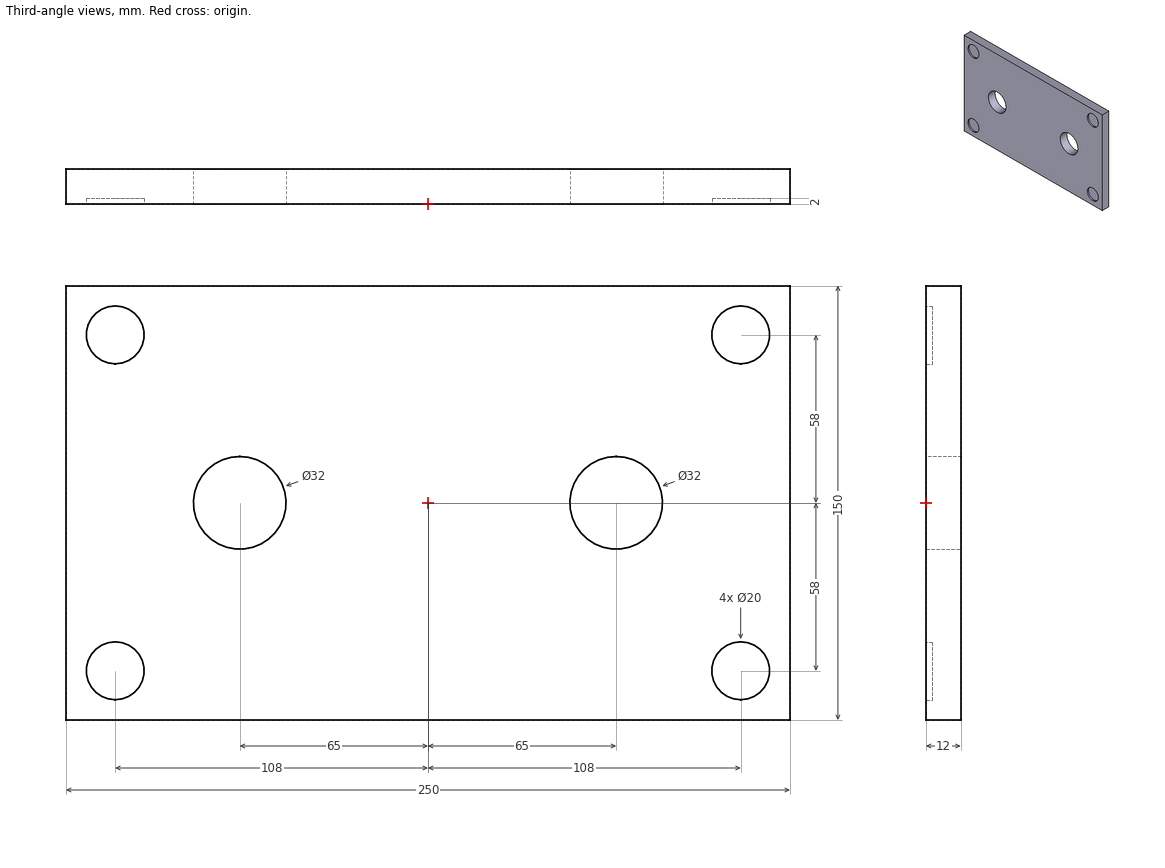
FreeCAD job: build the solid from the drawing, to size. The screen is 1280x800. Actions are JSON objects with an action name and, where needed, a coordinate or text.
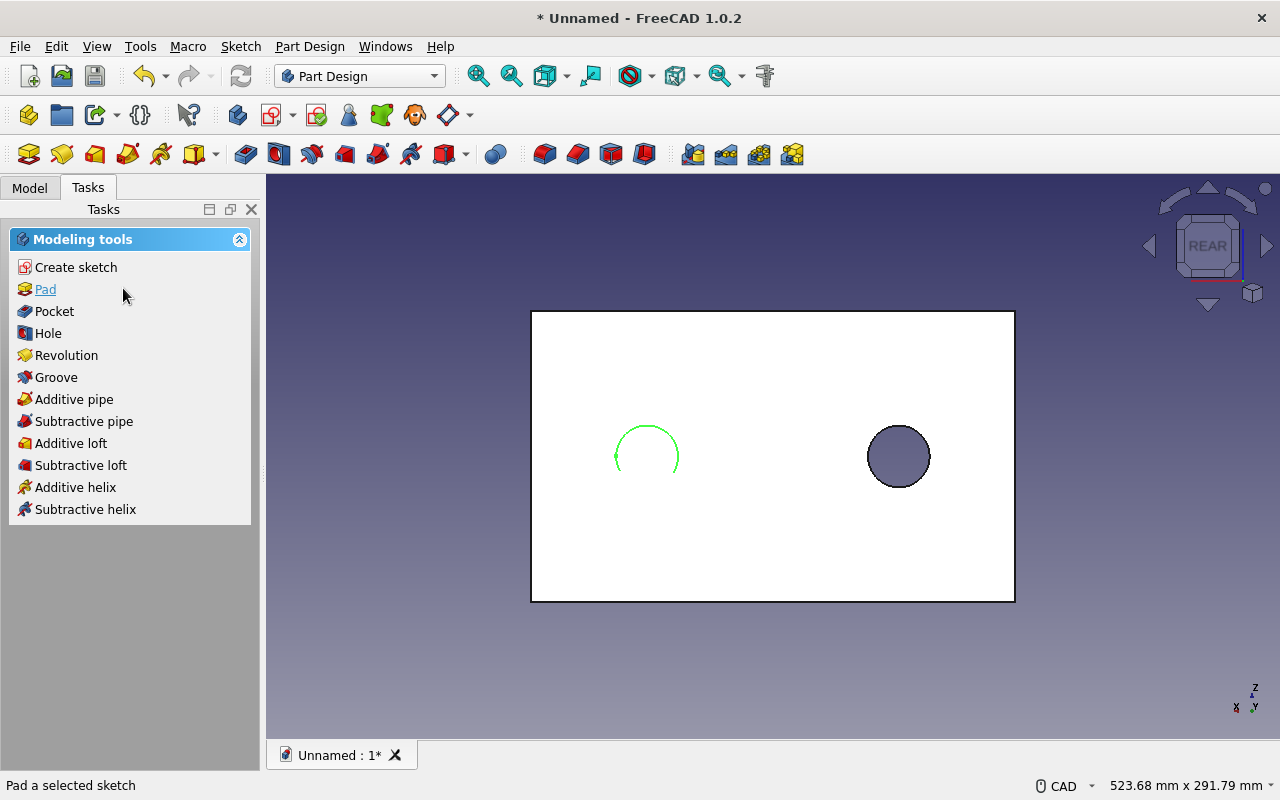
{"action": "left_click", "coordinate": [246, 154]}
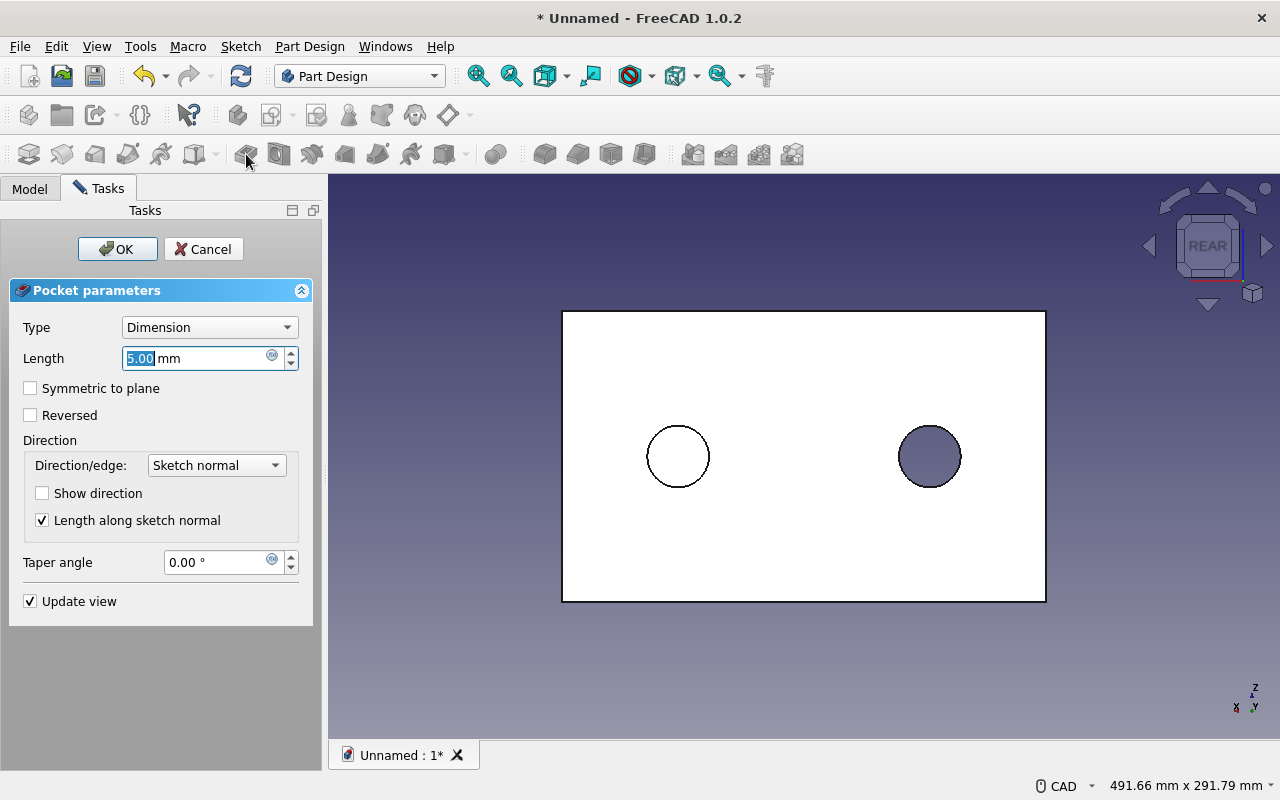
{"action": "left_click", "coordinate": [210, 328]}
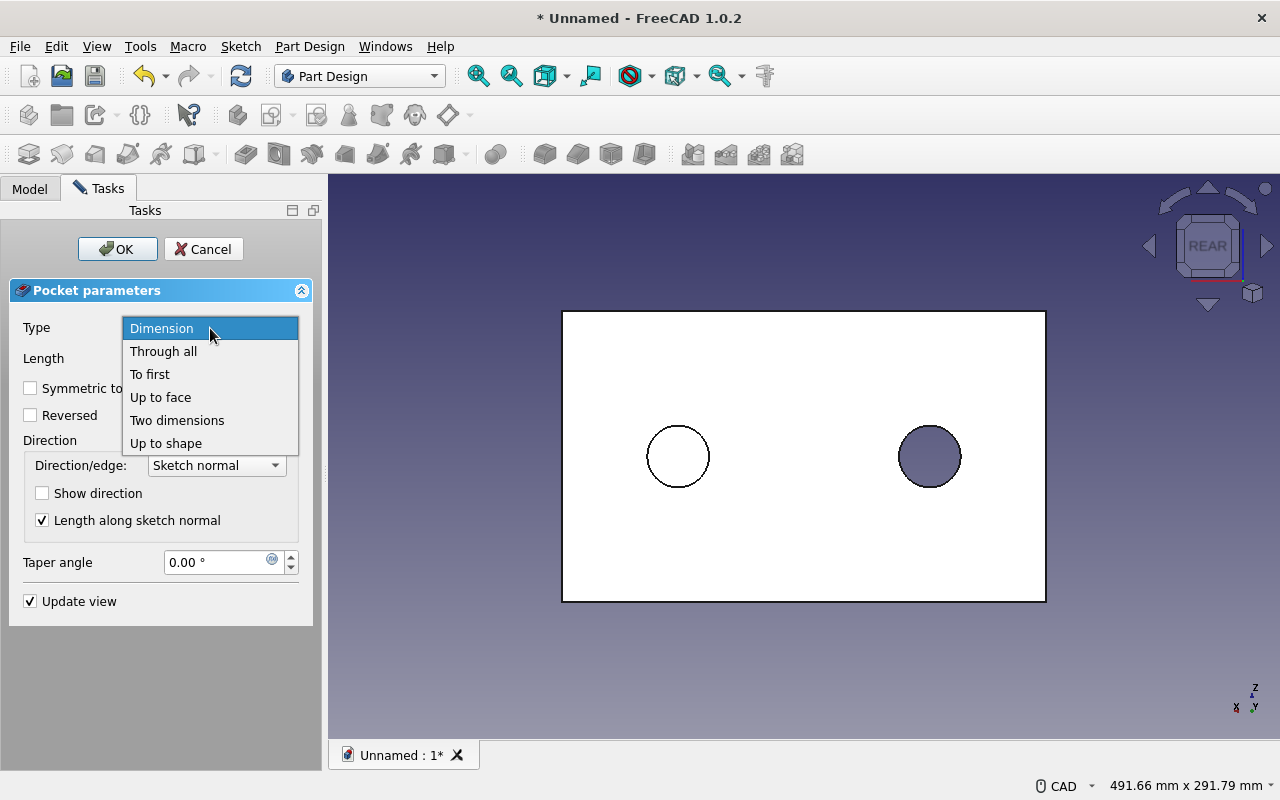
{"action": "left_click", "coordinate": [208, 374]}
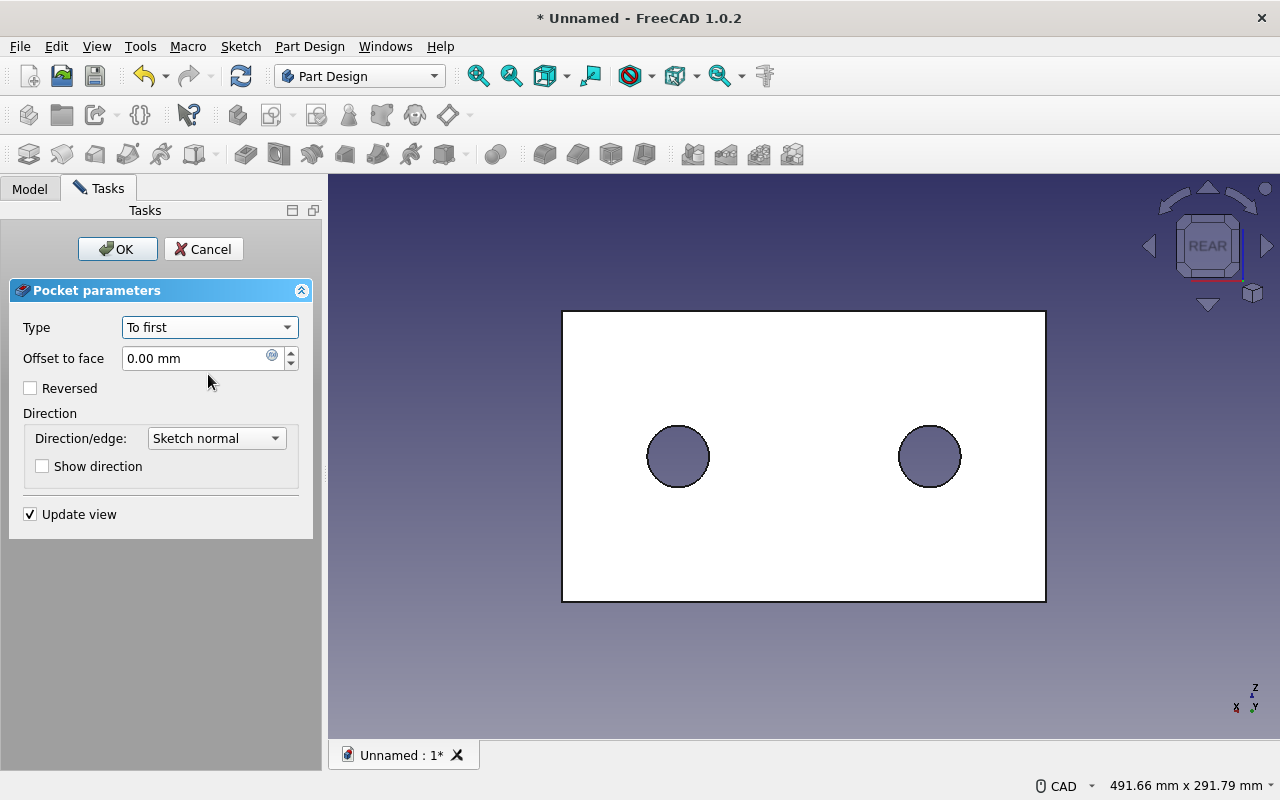
{"action": "left_click", "coordinate": [118, 249]}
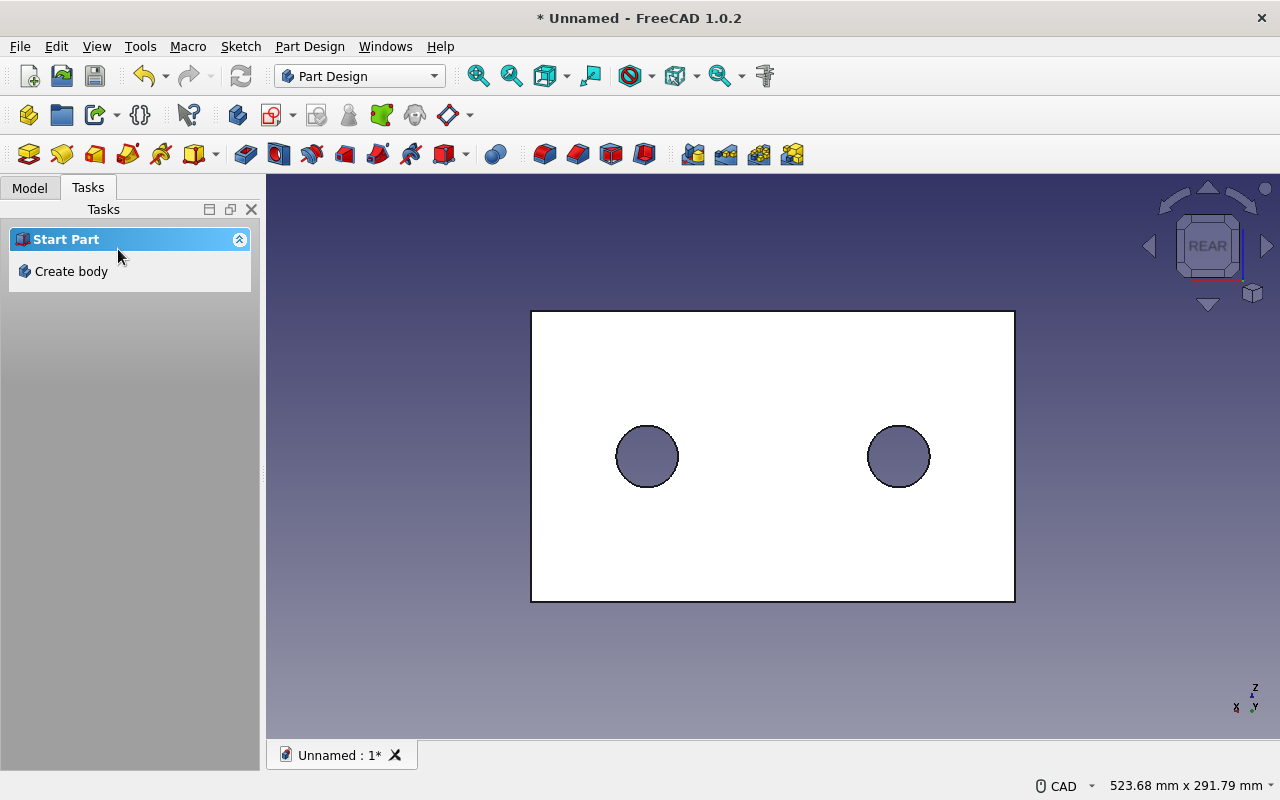
{"action": "key", "text": "0"}